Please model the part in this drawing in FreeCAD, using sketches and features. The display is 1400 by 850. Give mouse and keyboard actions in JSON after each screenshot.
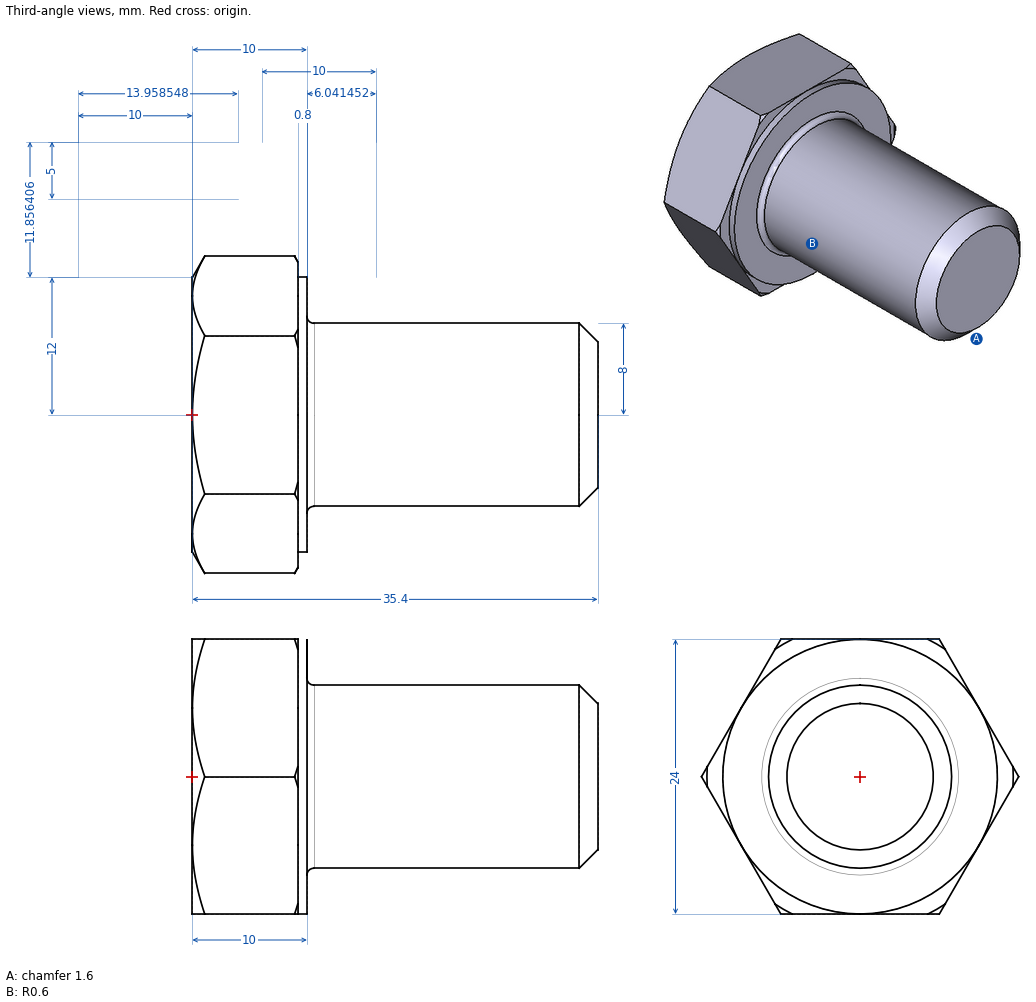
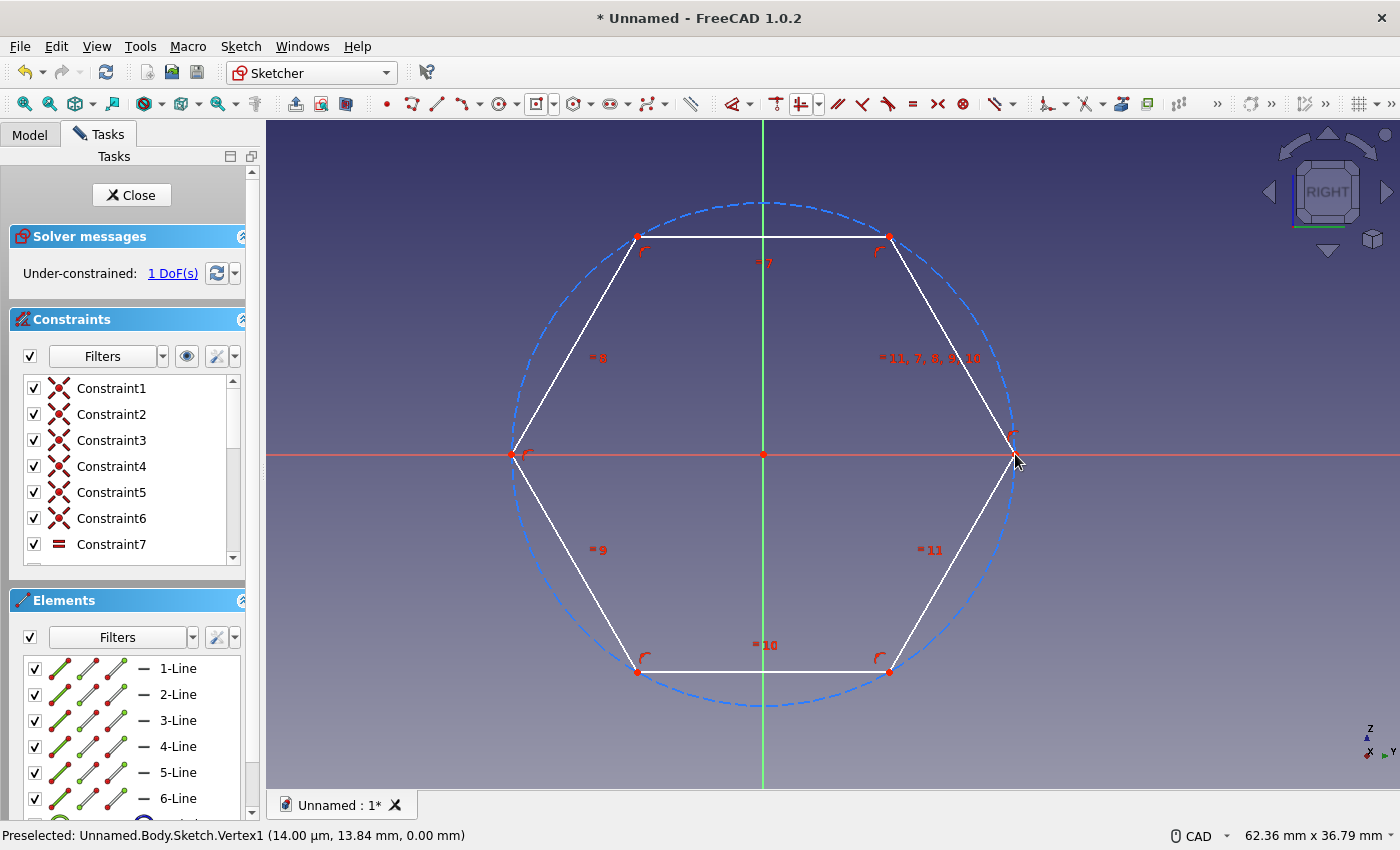
{"action": "left_click", "coordinate": [732, 104]}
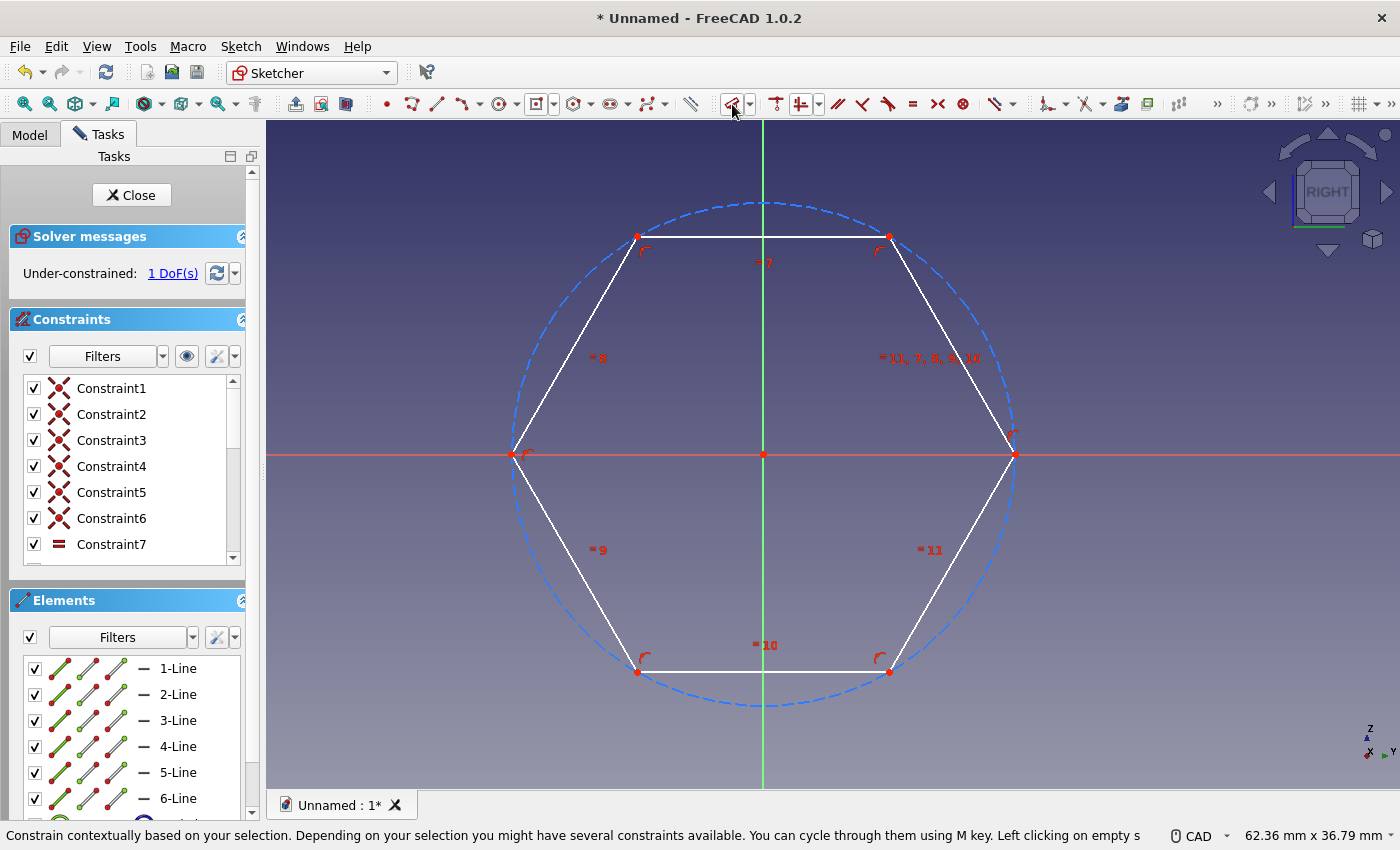
{"action": "left_click", "coordinate": [638, 672]}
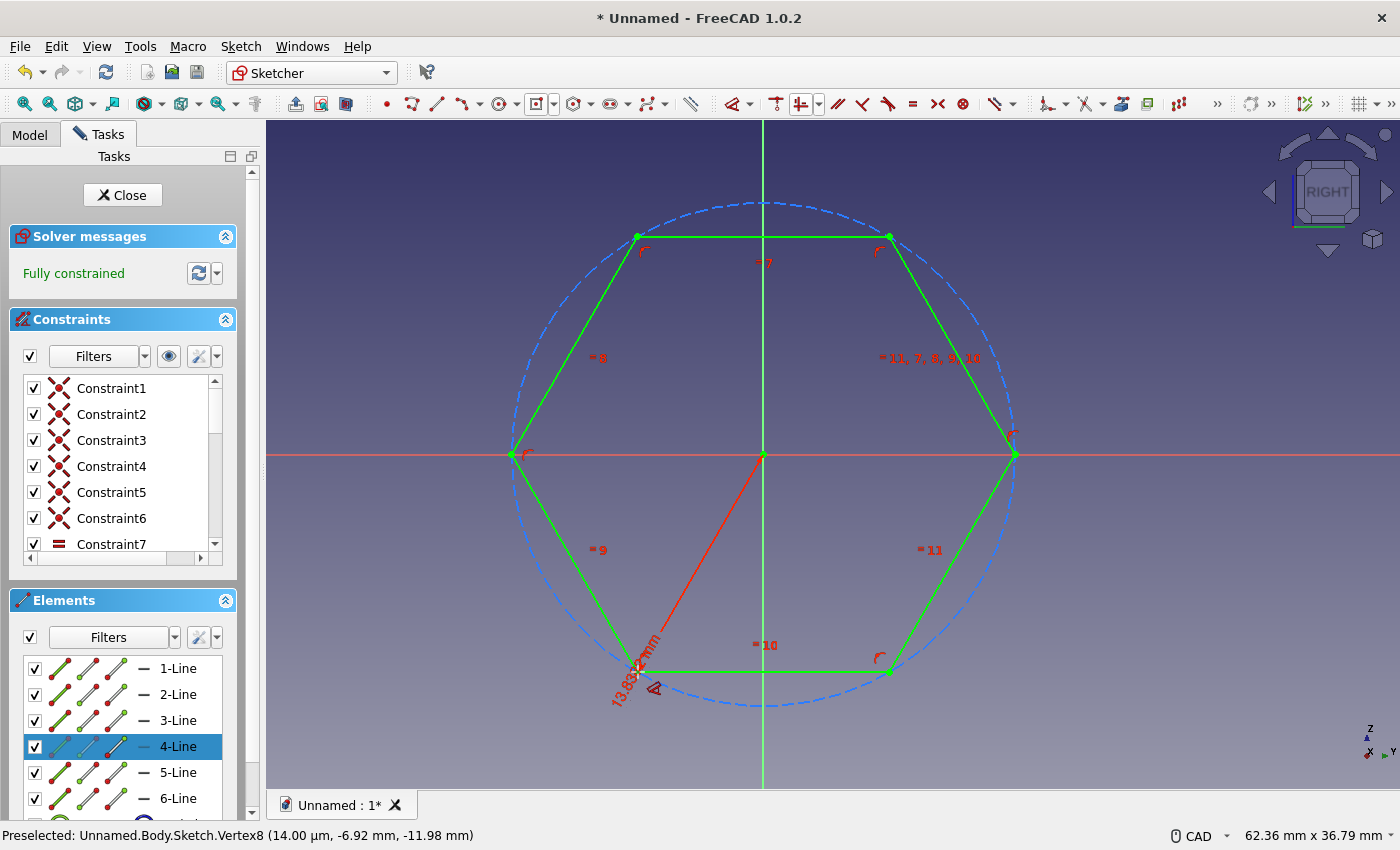
{"action": "left_click", "coordinate": [889, 237]}
{"action": "left_click", "coordinate": [923, 354]}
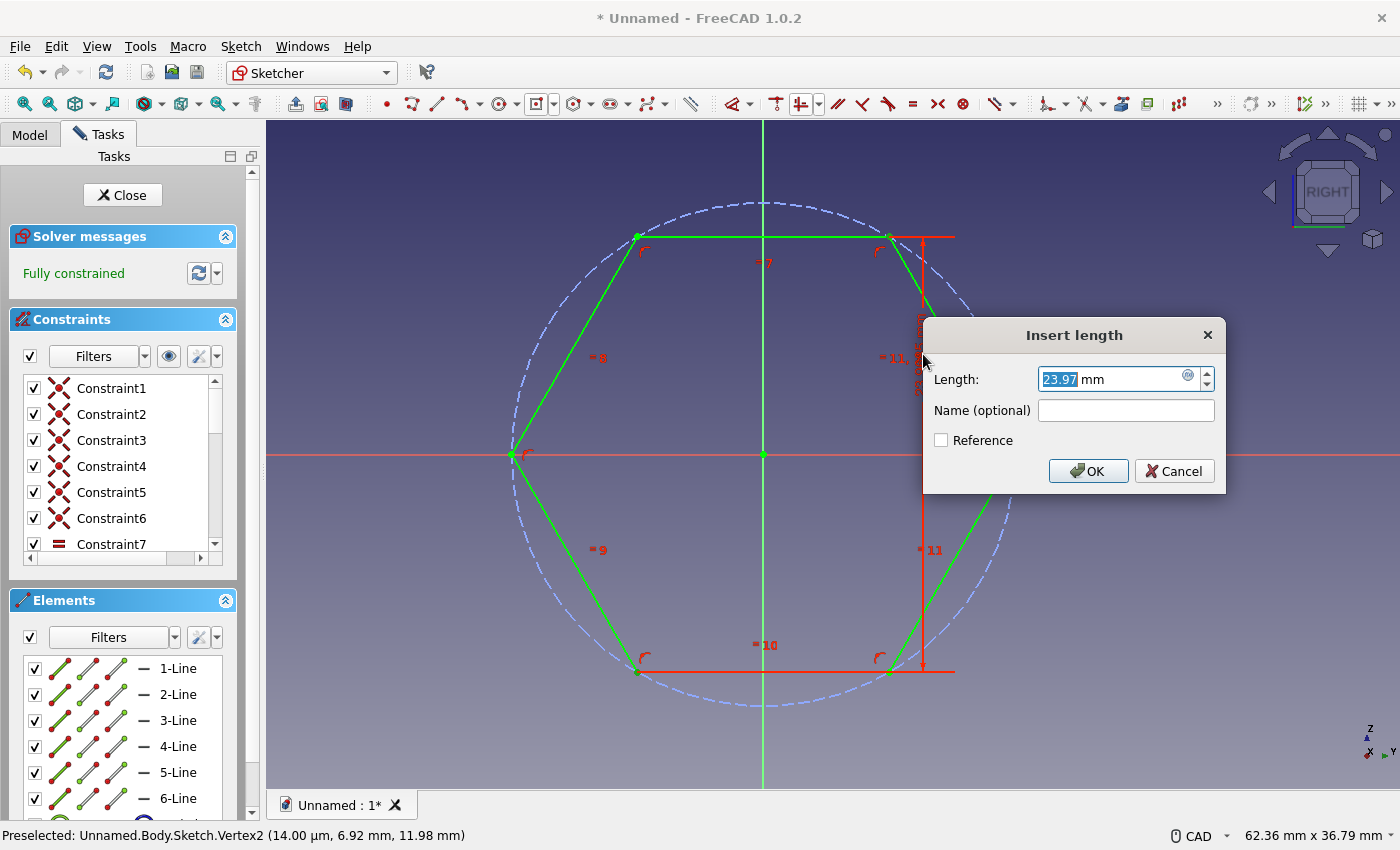
{"action": "type", "text": "24"}
{"action": "key", "text": "Return"}
{"action": "key", "text": "Escape"}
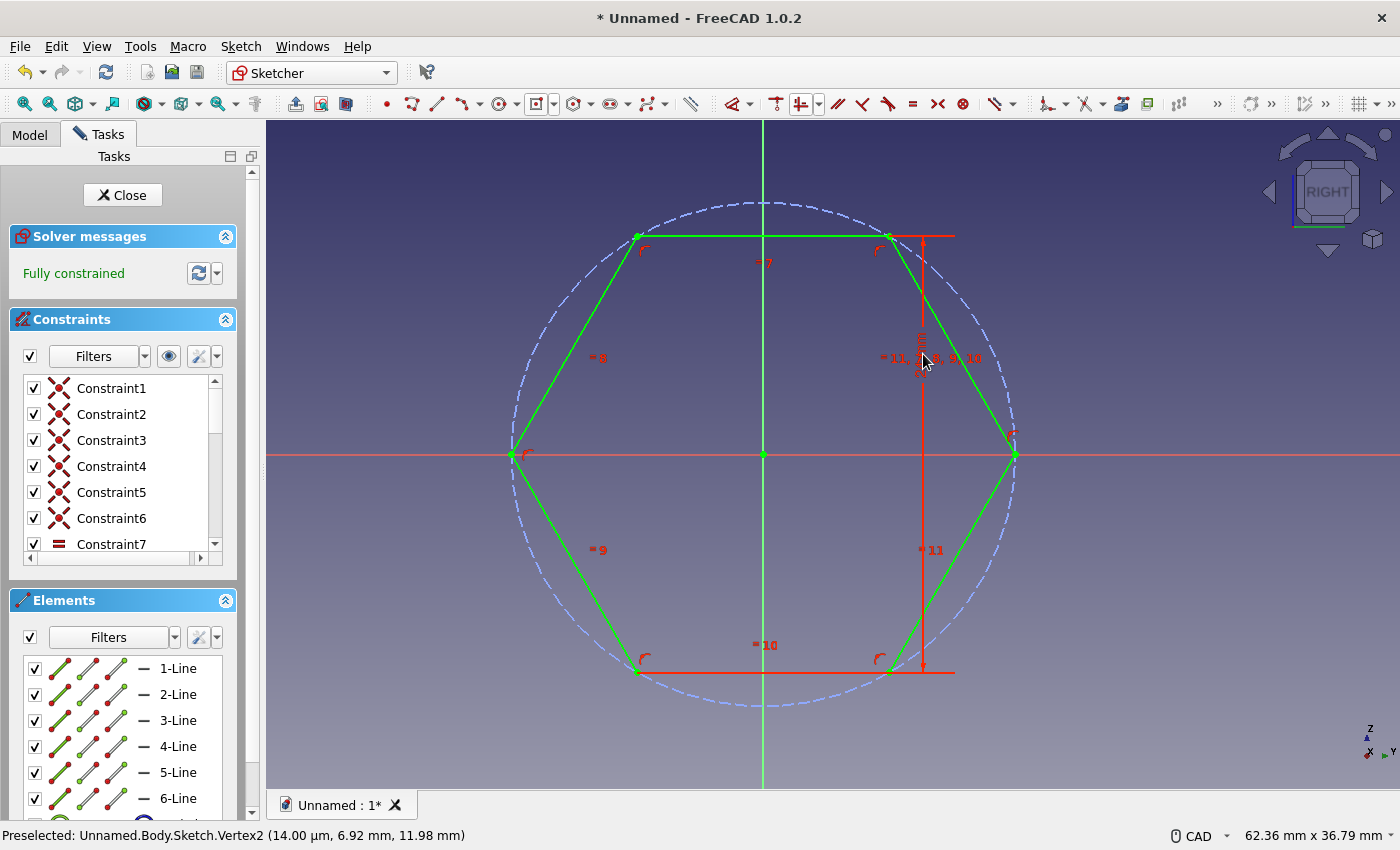
{"action": "left_click", "coordinate": [123, 195]}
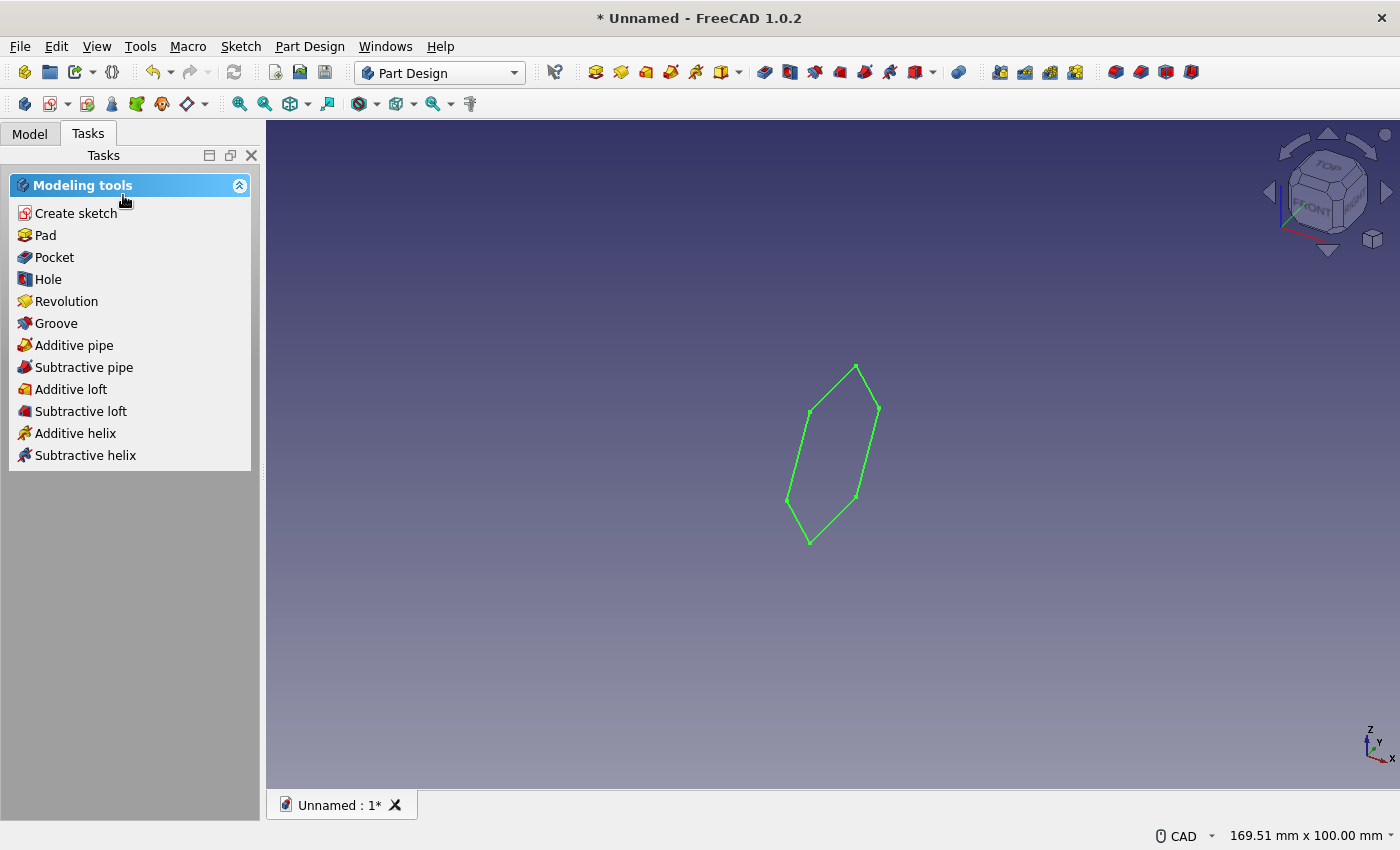
{"action": "left_click", "coordinate": [596, 72]}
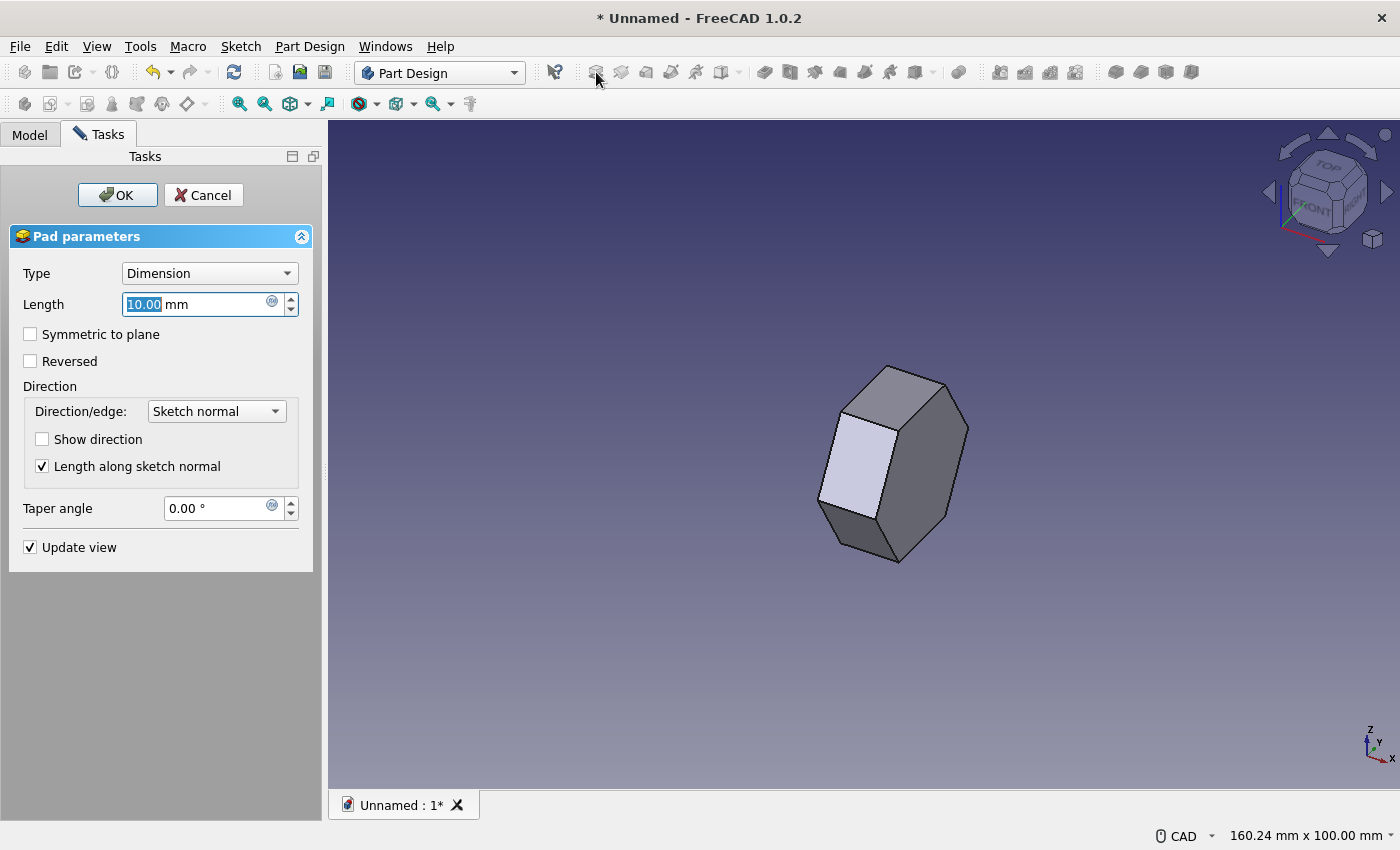
{"action": "type", "text": "10"}
{"action": "key", "text": "Tab"}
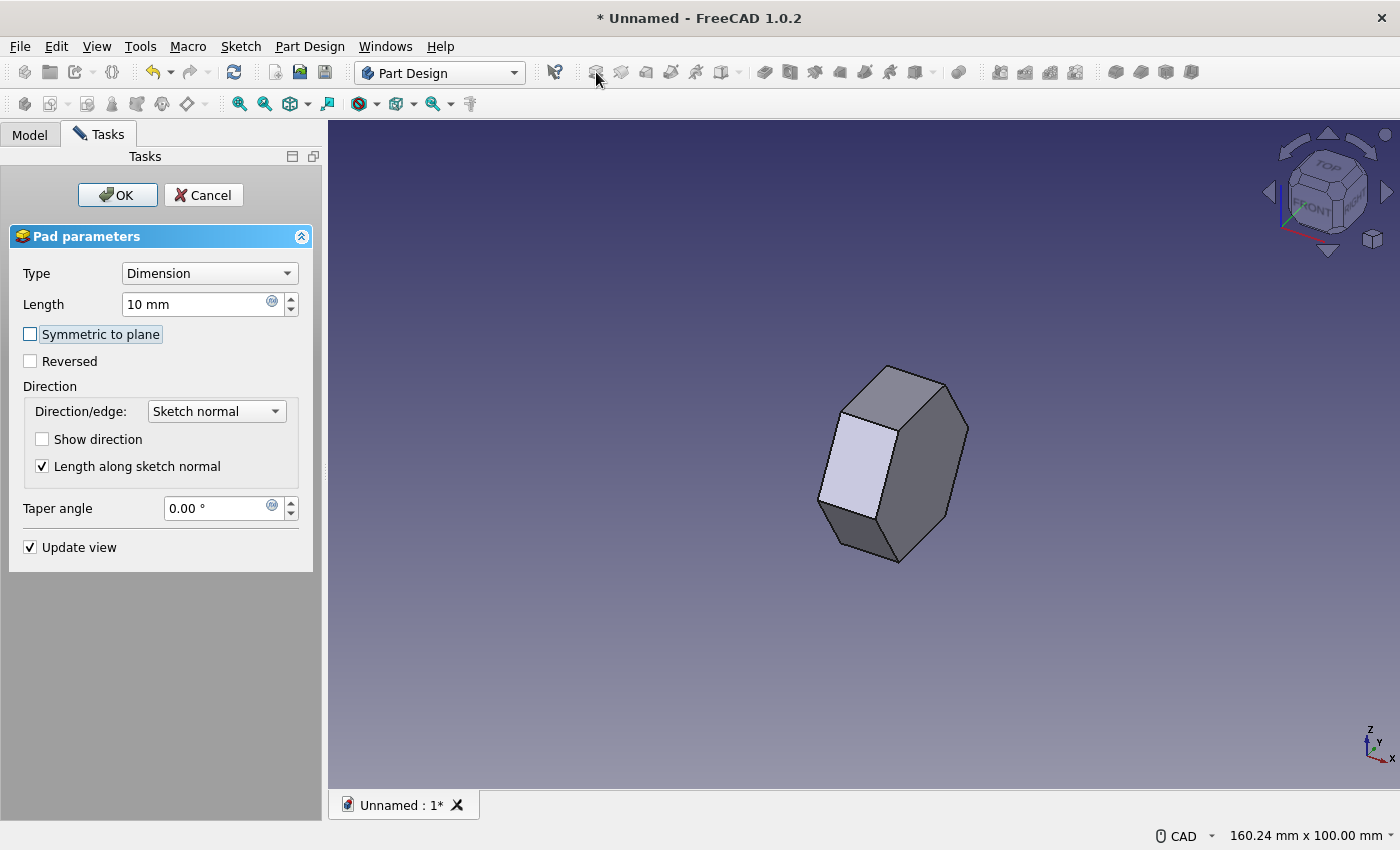
{"action": "left_click", "coordinate": [118, 195]}